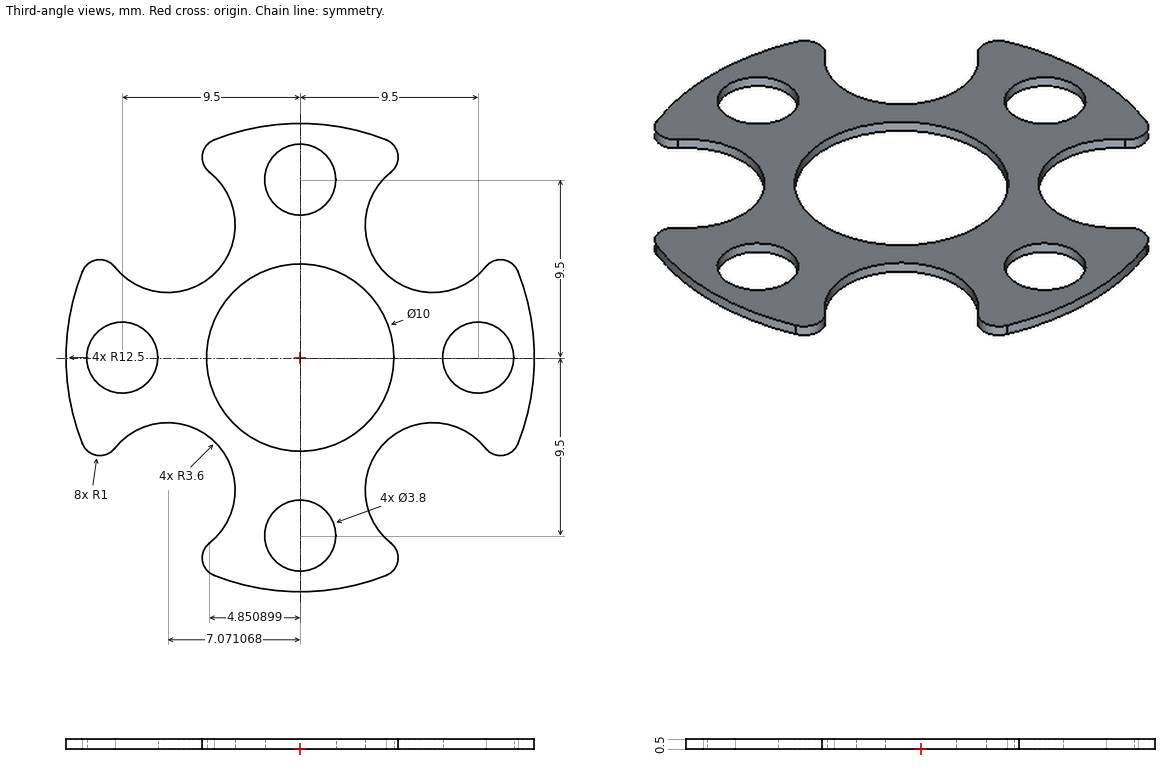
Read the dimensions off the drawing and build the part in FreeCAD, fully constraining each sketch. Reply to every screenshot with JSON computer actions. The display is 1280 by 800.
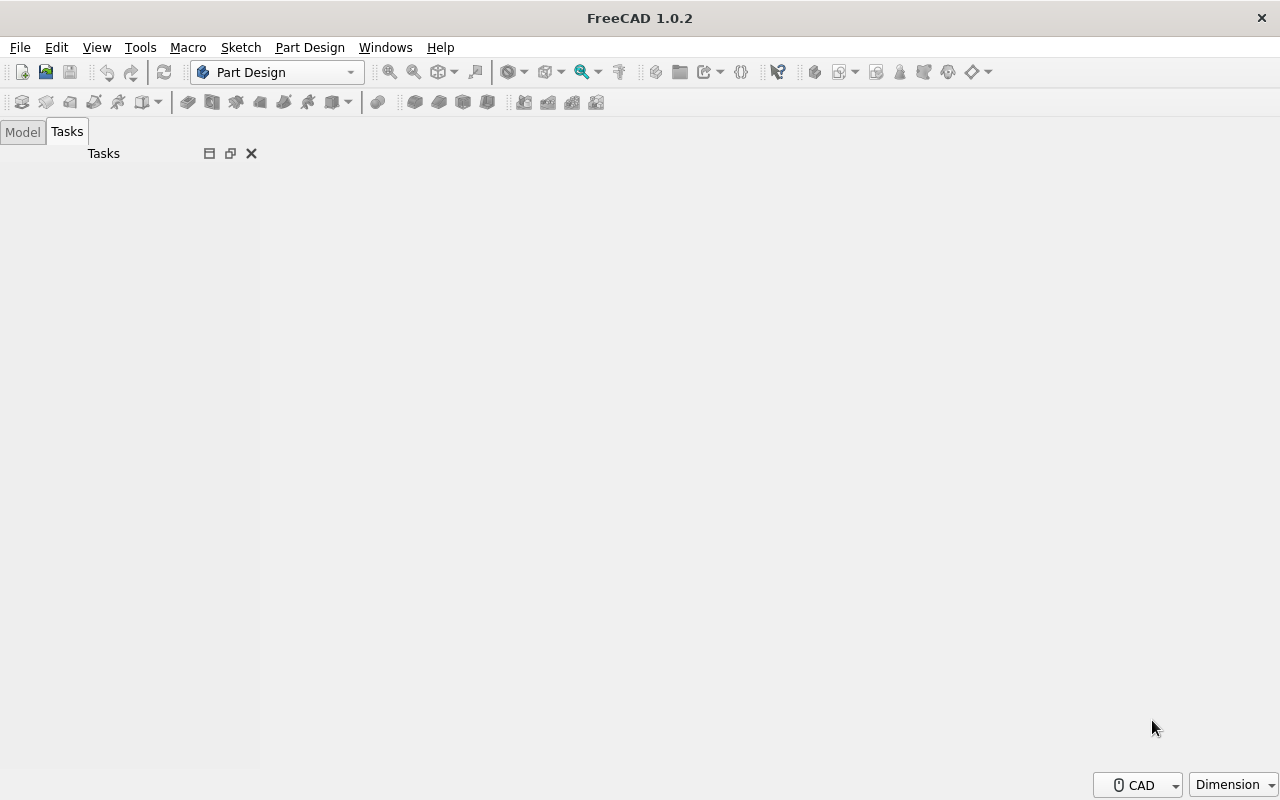
{"action": "key", "text": "ctrl+n"}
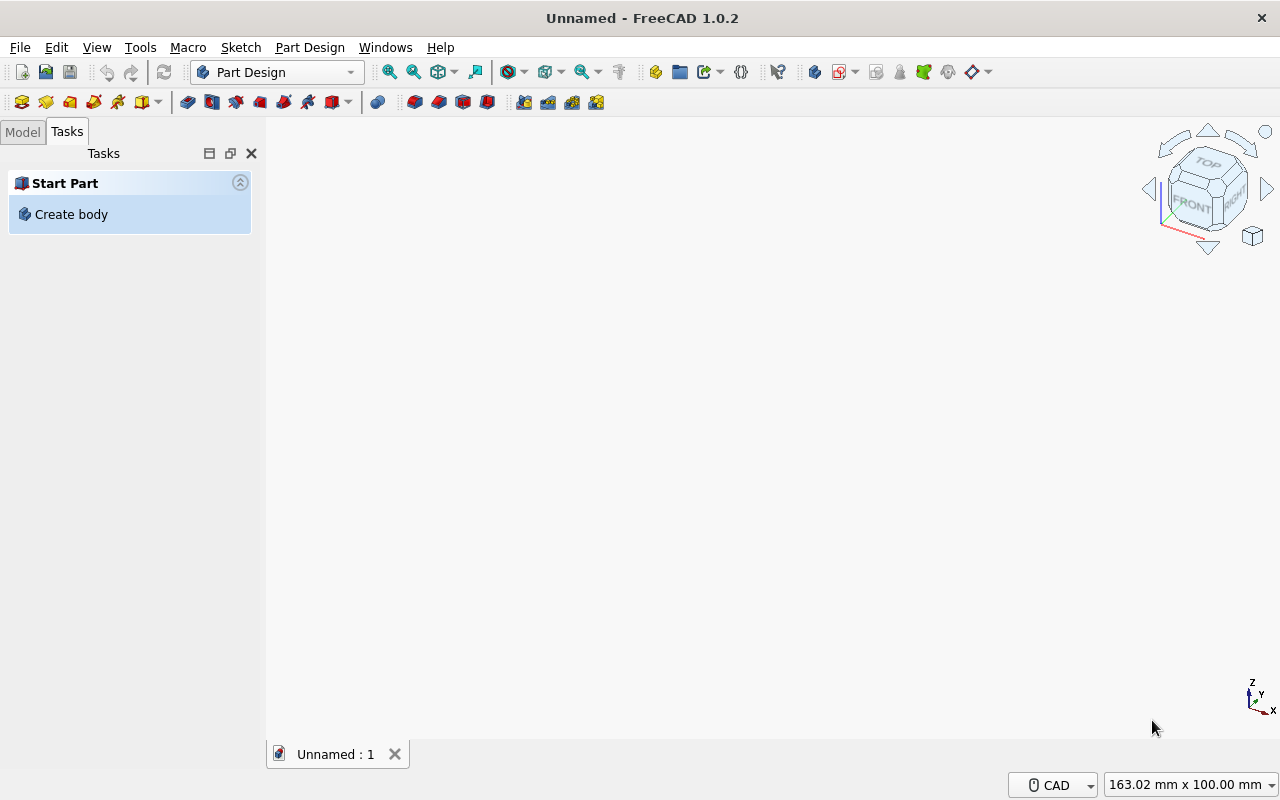
{"action": "left_click", "coordinate": [840, 72]}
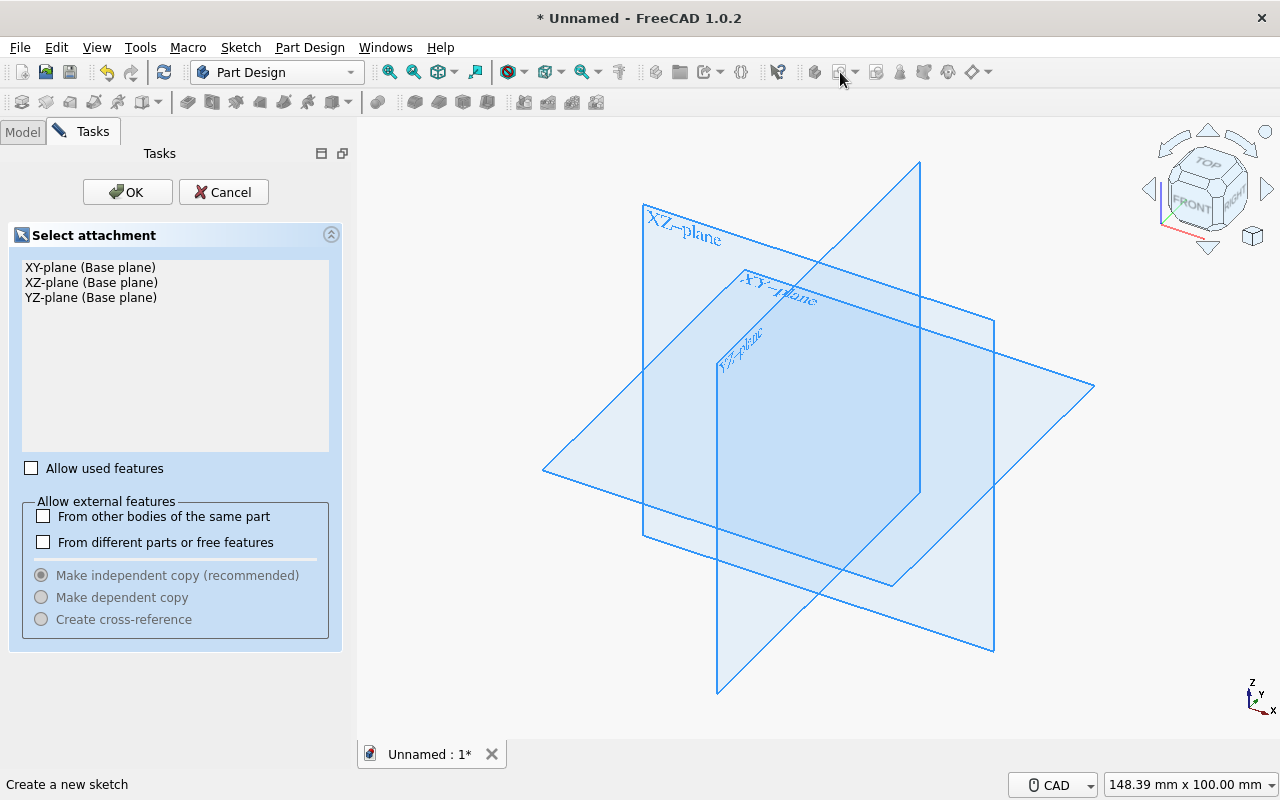
{"action": "left_click", "coordinate": [82, 268]}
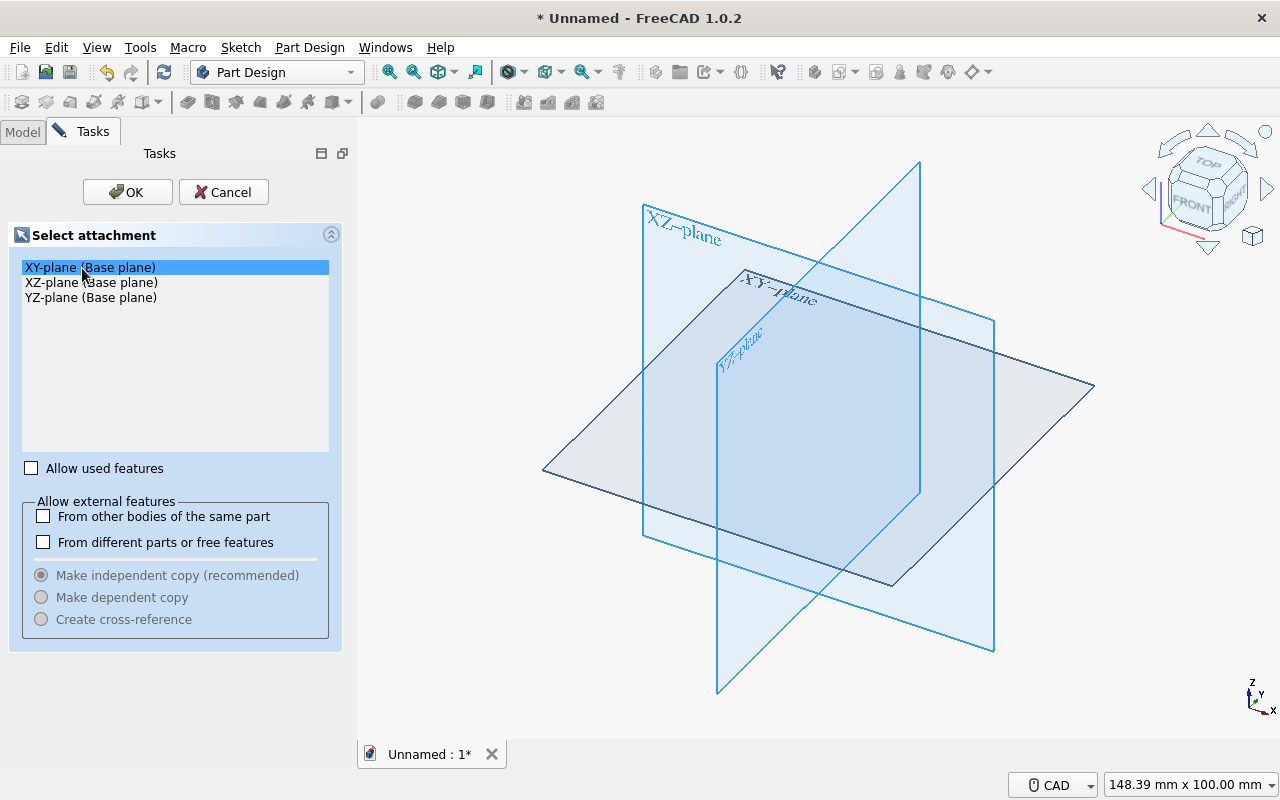
{"action": "left_click", "coordinate": [128, 192]}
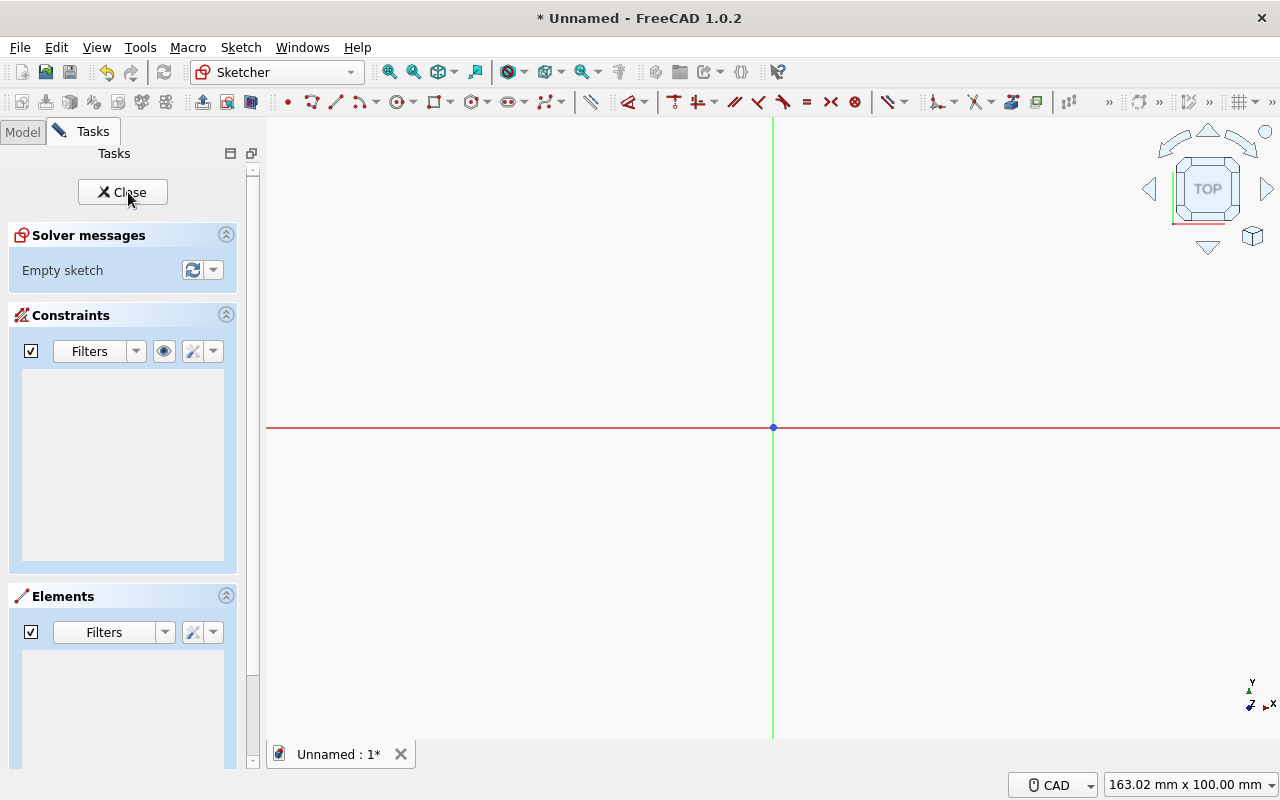
{"action": "scroll", "coordinate": [813, 428], "scroll_direction": "up", "scroll_amount": 5}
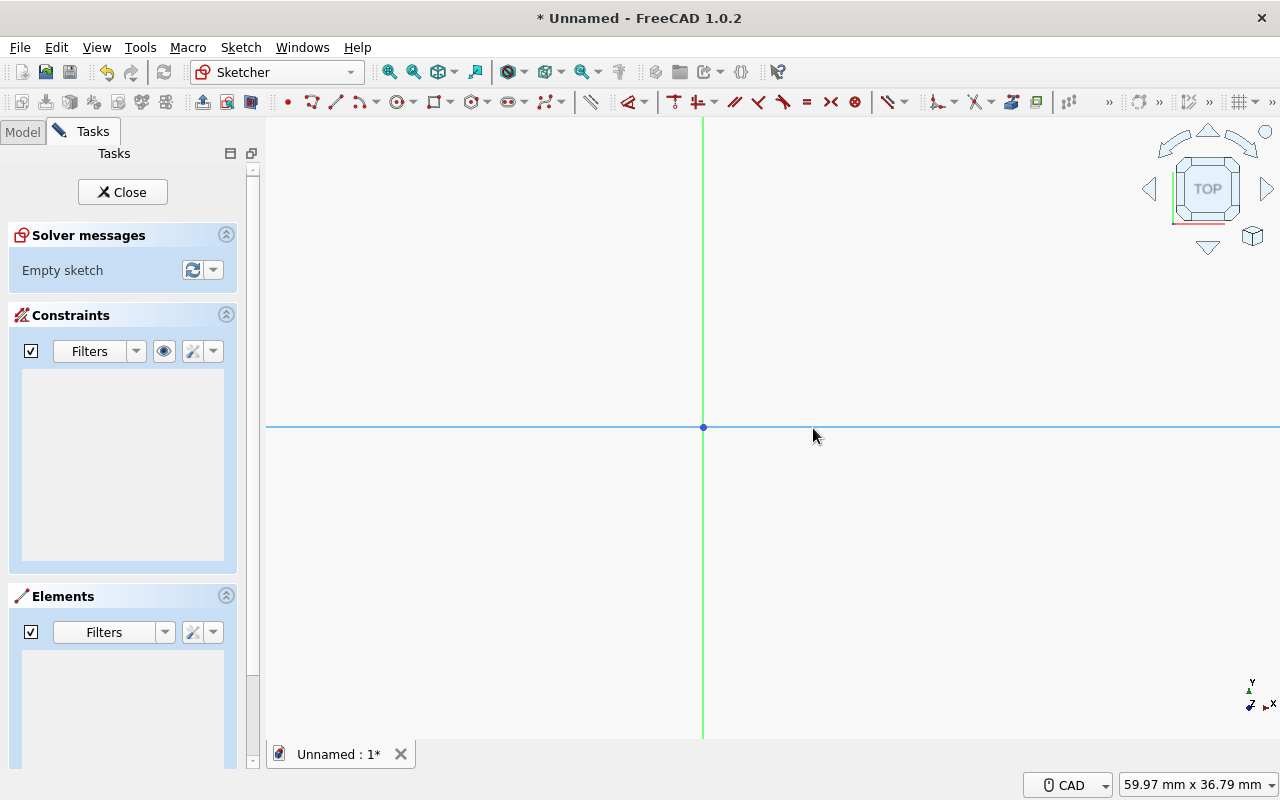
{"action": "key", "text": "g 3 a"}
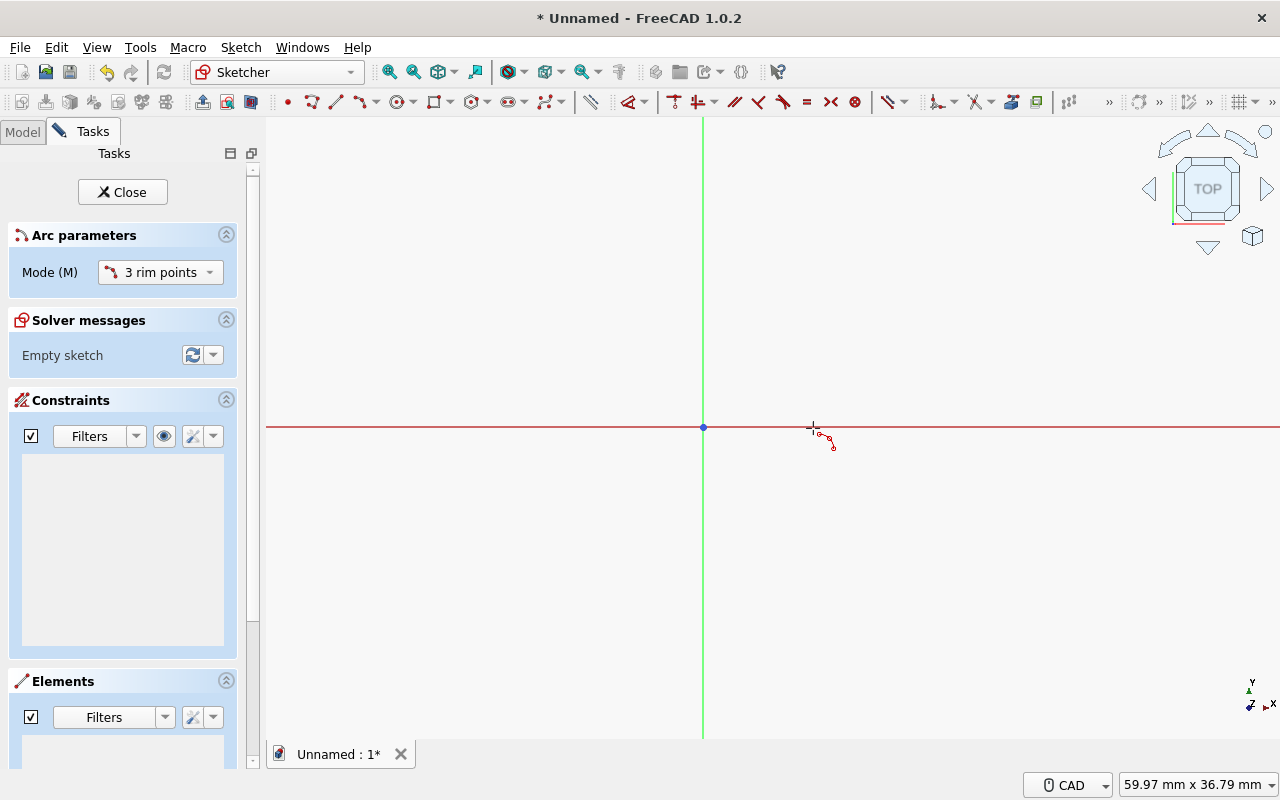
{"action": "left_click", "coordinate": [536, 509]}
{"action": "left_click", "coordinate": [621, 595]}
{"action": "left_click", "coordinate": [627, 504]}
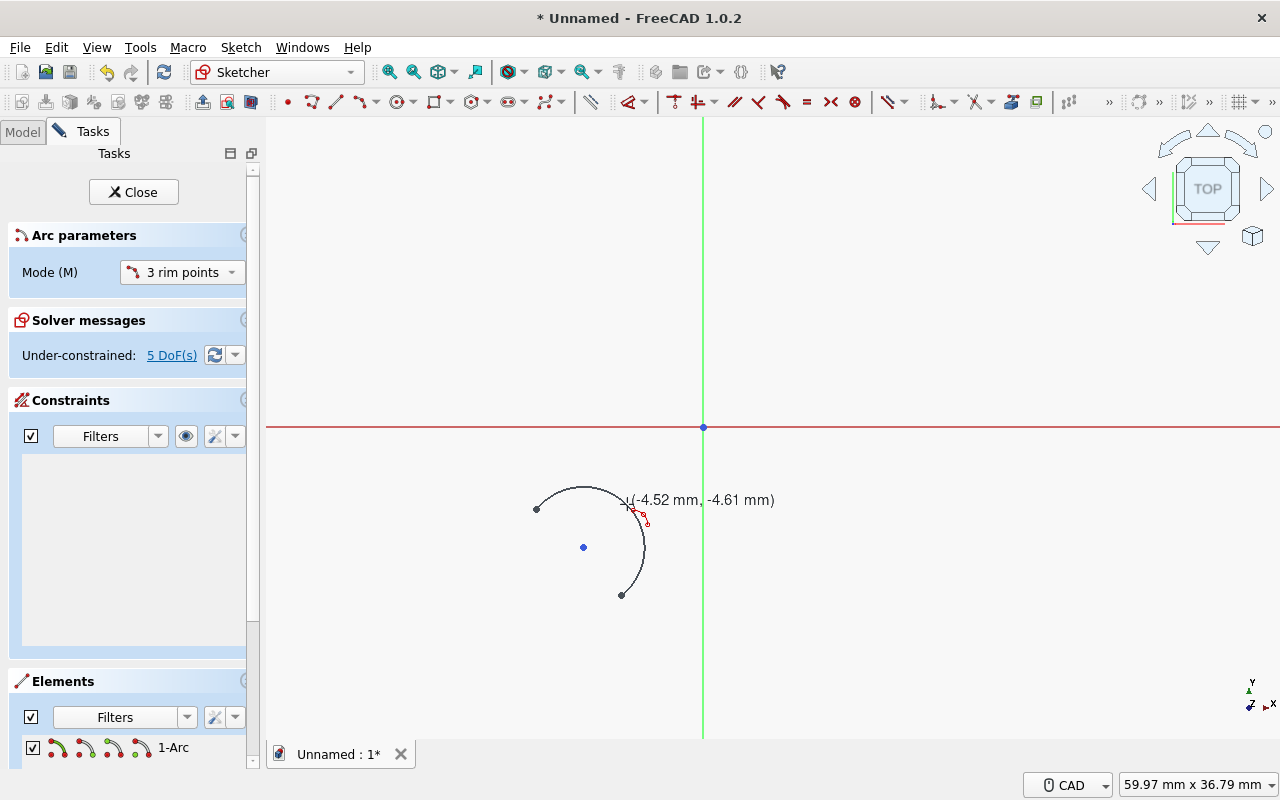
{"action": "left_click", "coordinate": [621, 596]}
{"action": "left_click", "coordinate": [626, 624]}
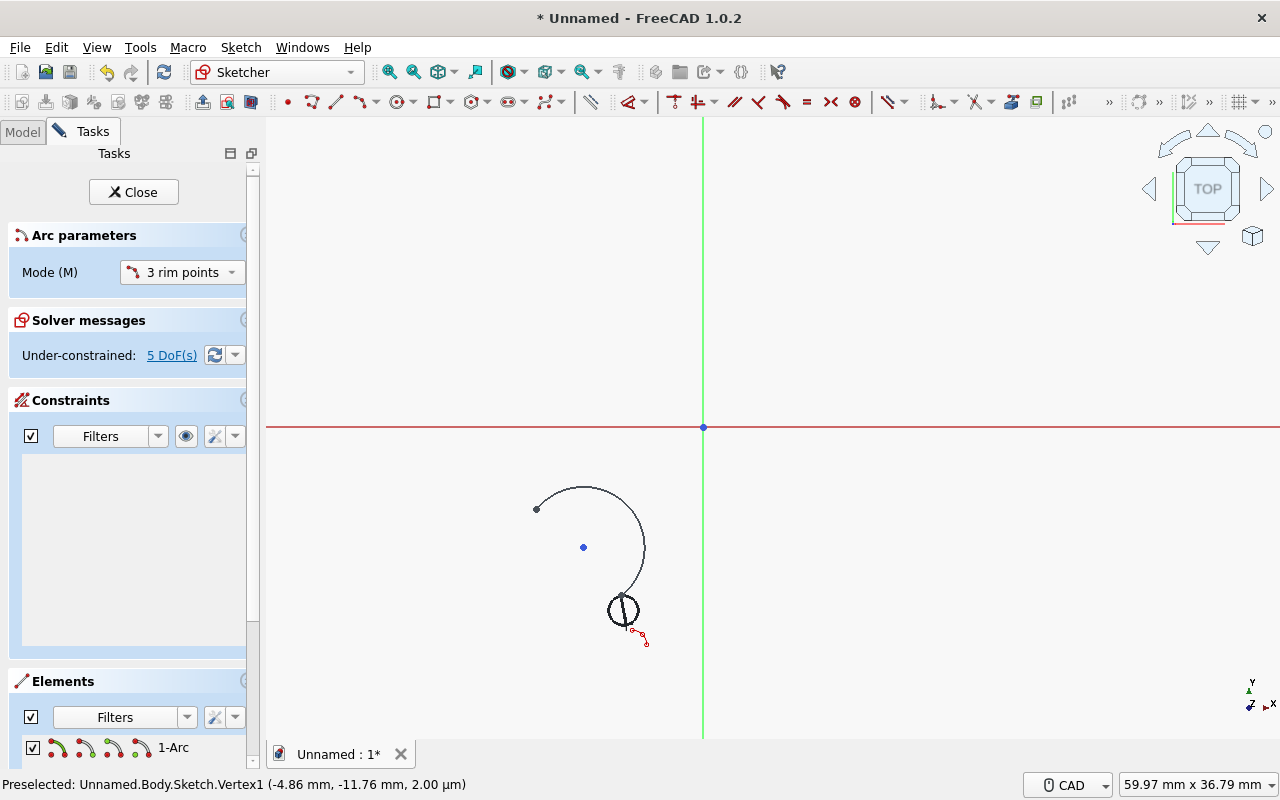
{"action": "scroll", "coordinate": [615, 610], "scroll_direction": "up", "scroll_amount": 4}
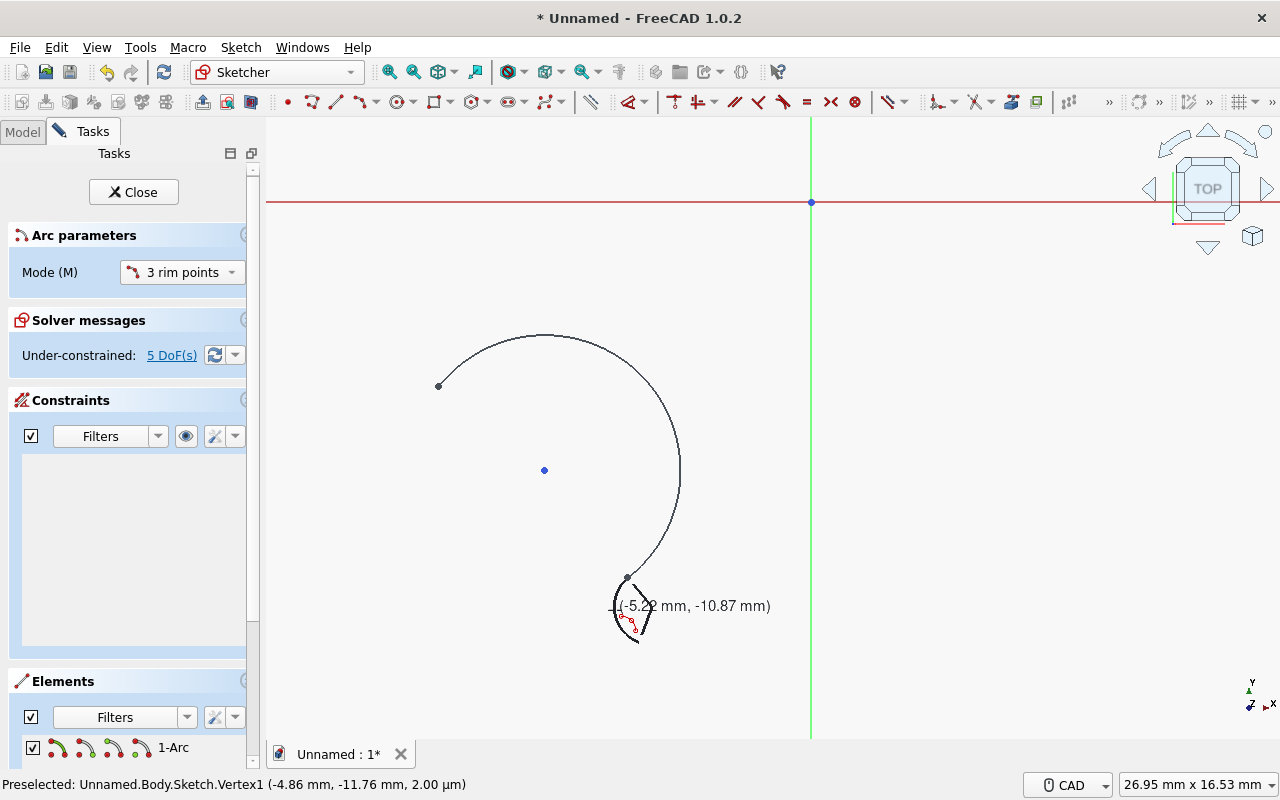
{"action": "left_click", "coordinate": [615, 610]}